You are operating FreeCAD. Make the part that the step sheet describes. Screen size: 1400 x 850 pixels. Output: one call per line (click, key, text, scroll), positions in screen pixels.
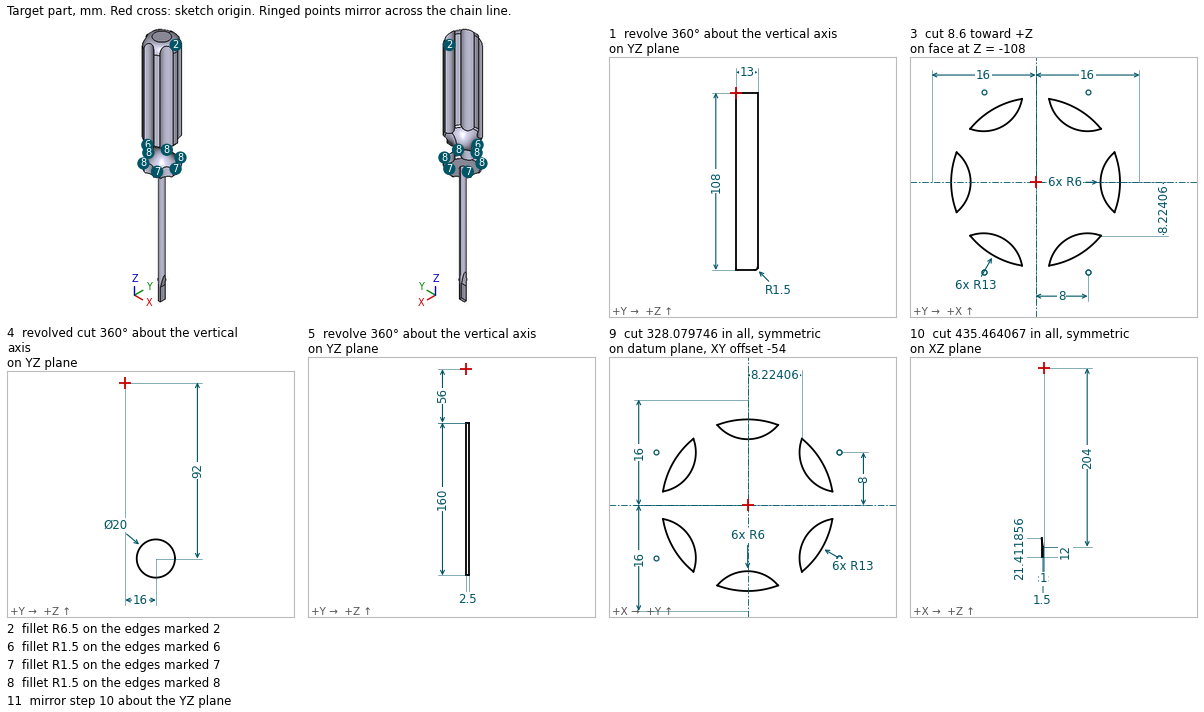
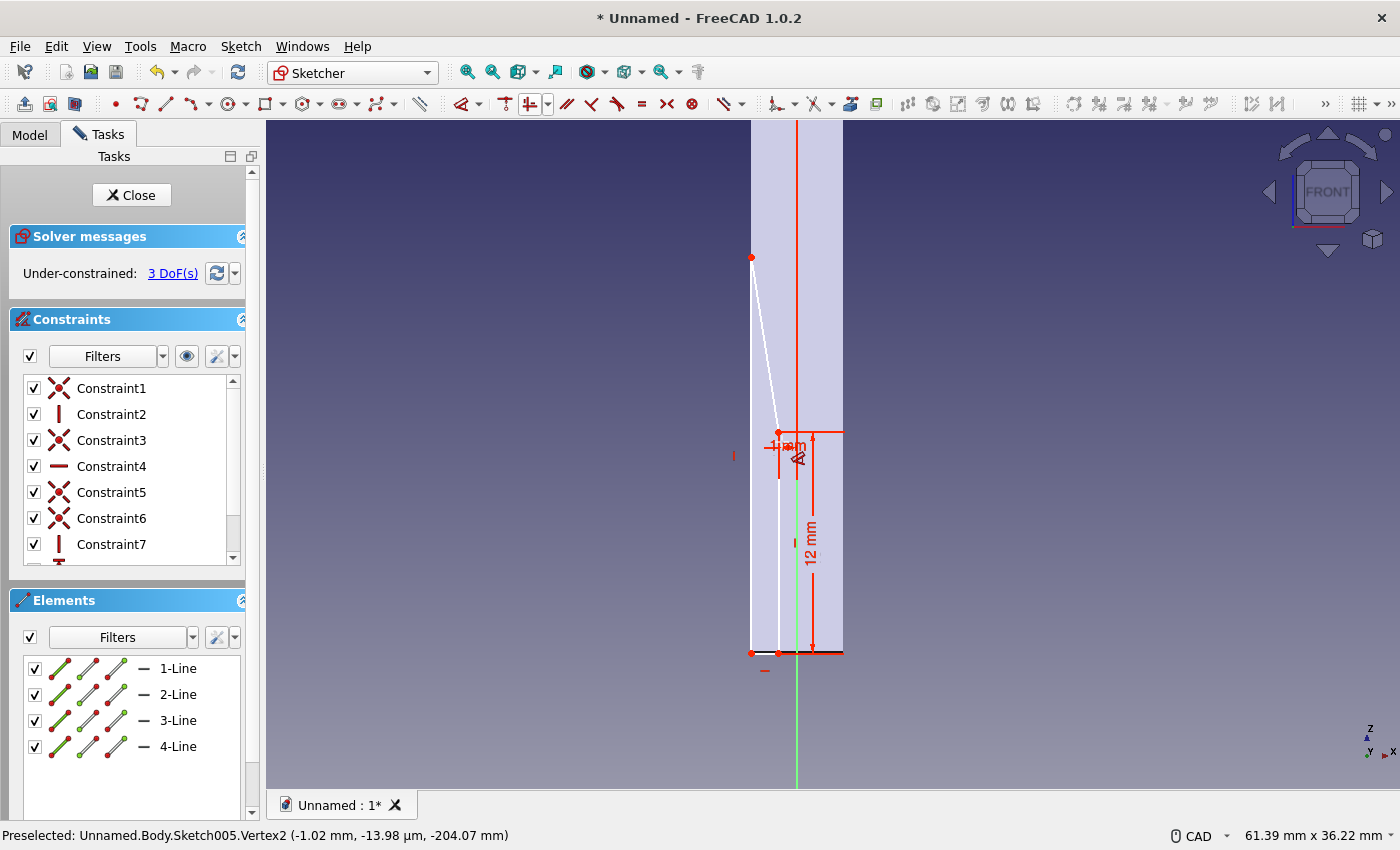
scroll(771, 654, up, 3)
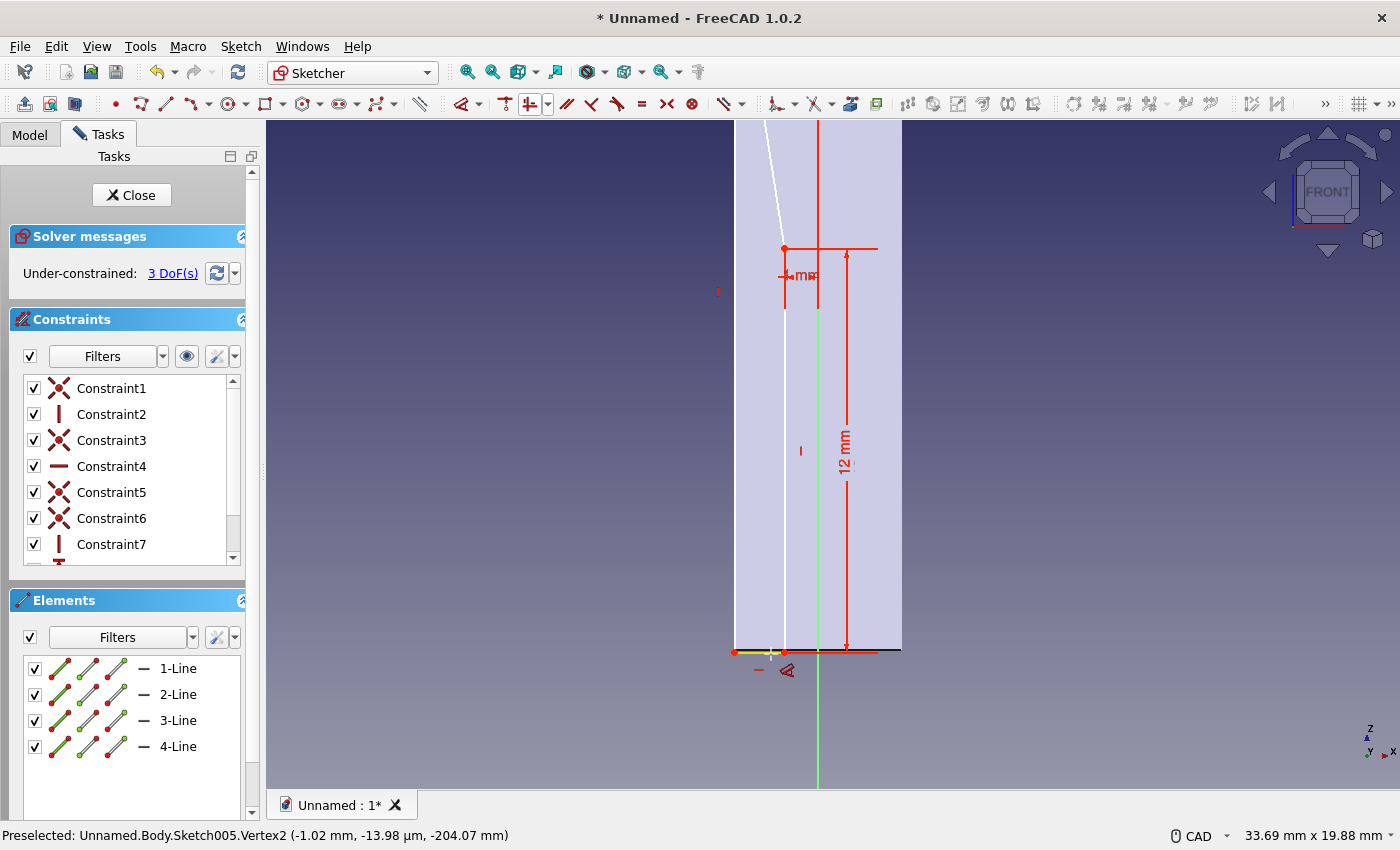
click(770, 653)
click(760, 687)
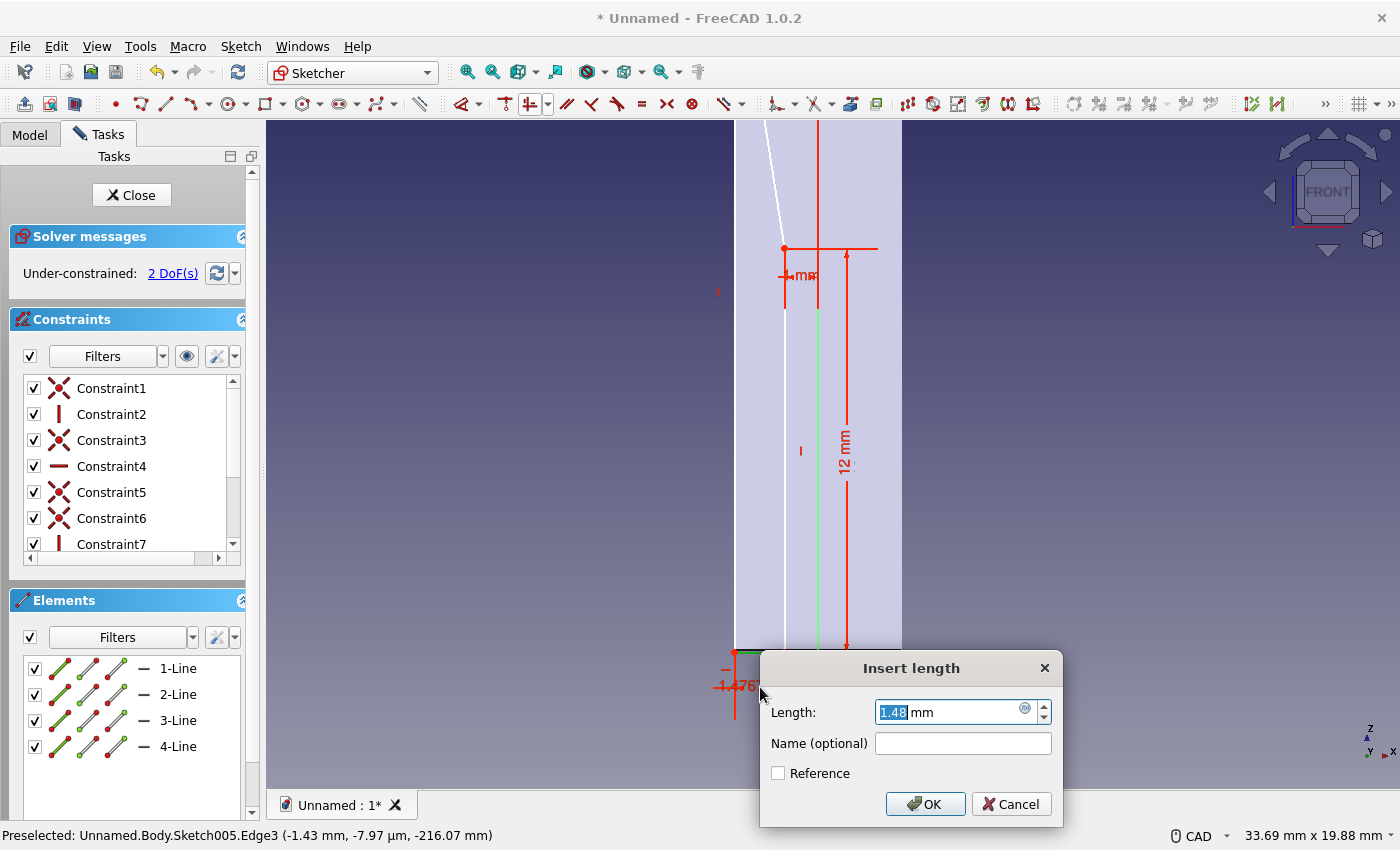
text(1.5)
key(Return)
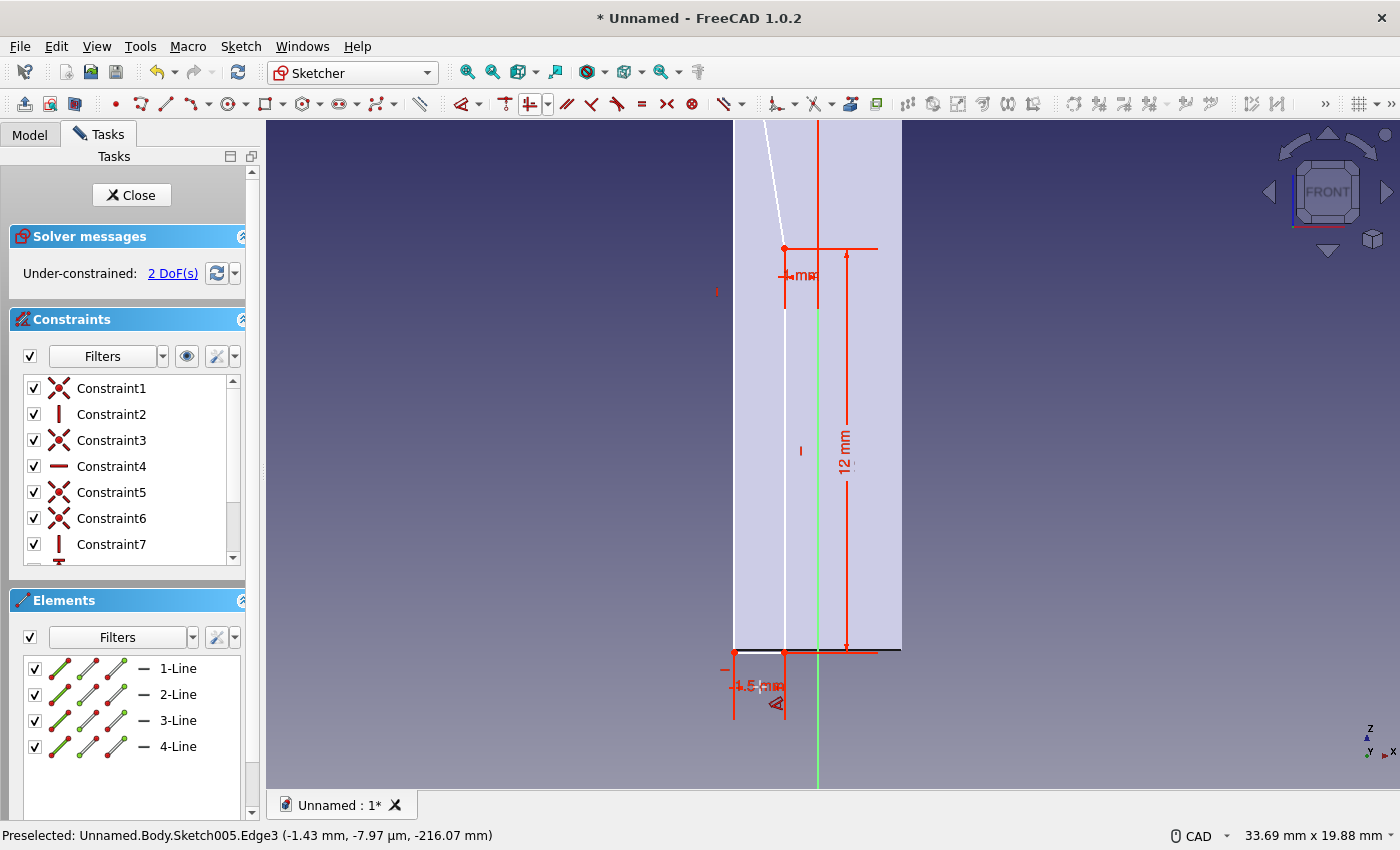
click(785, 249)
click(852, 198)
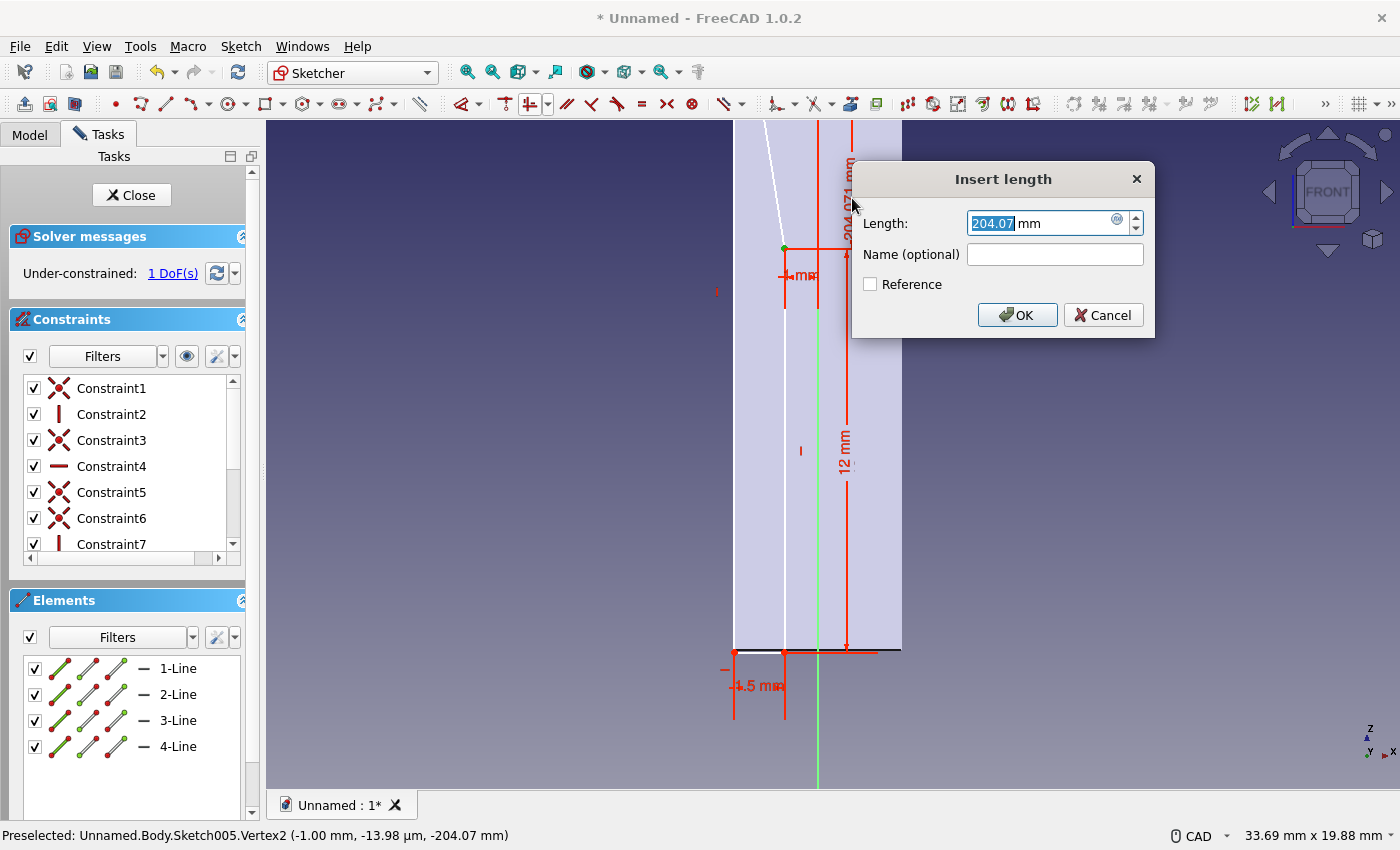
text(204)
key(Return)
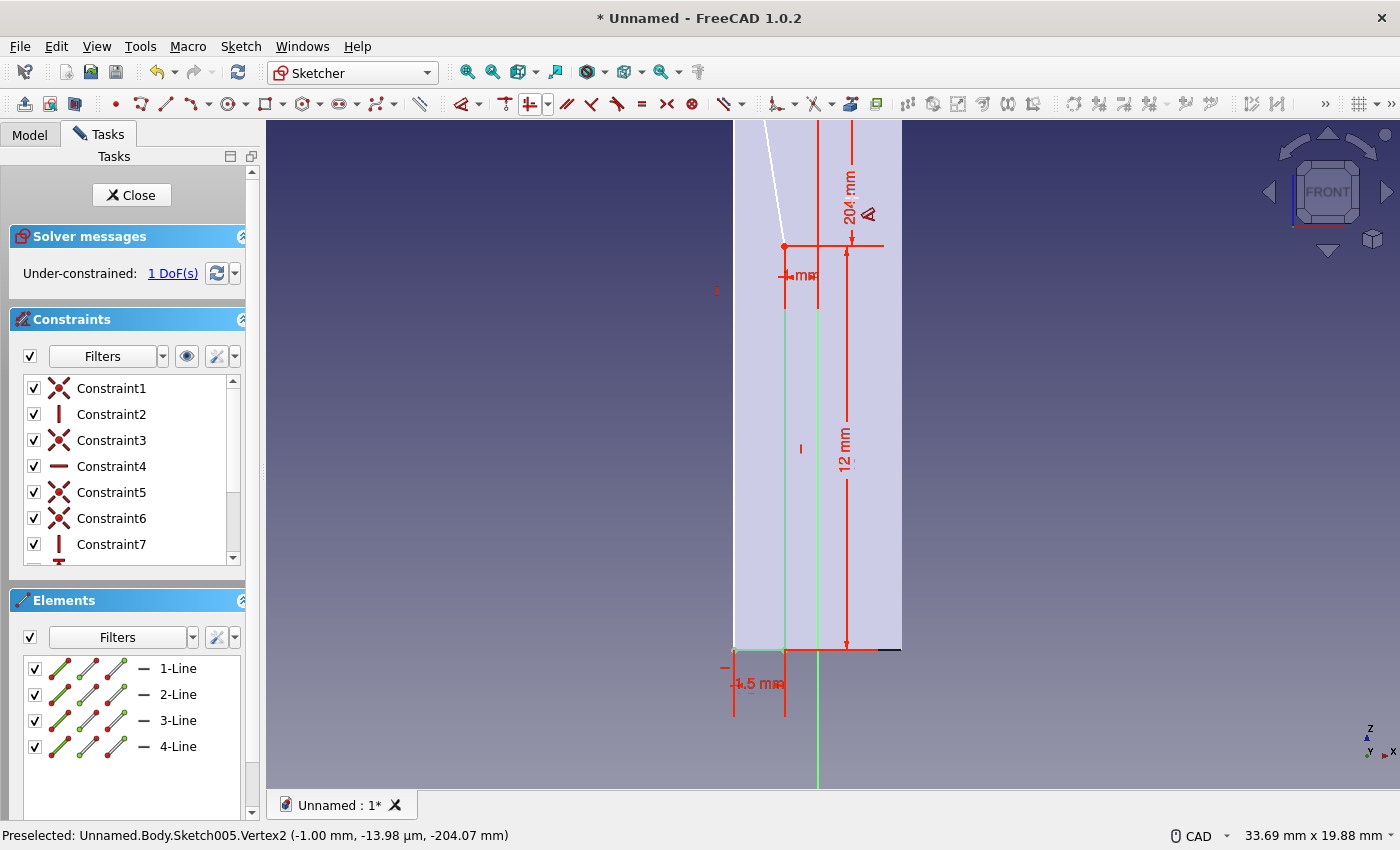
click(734, 435)
click(700, 399)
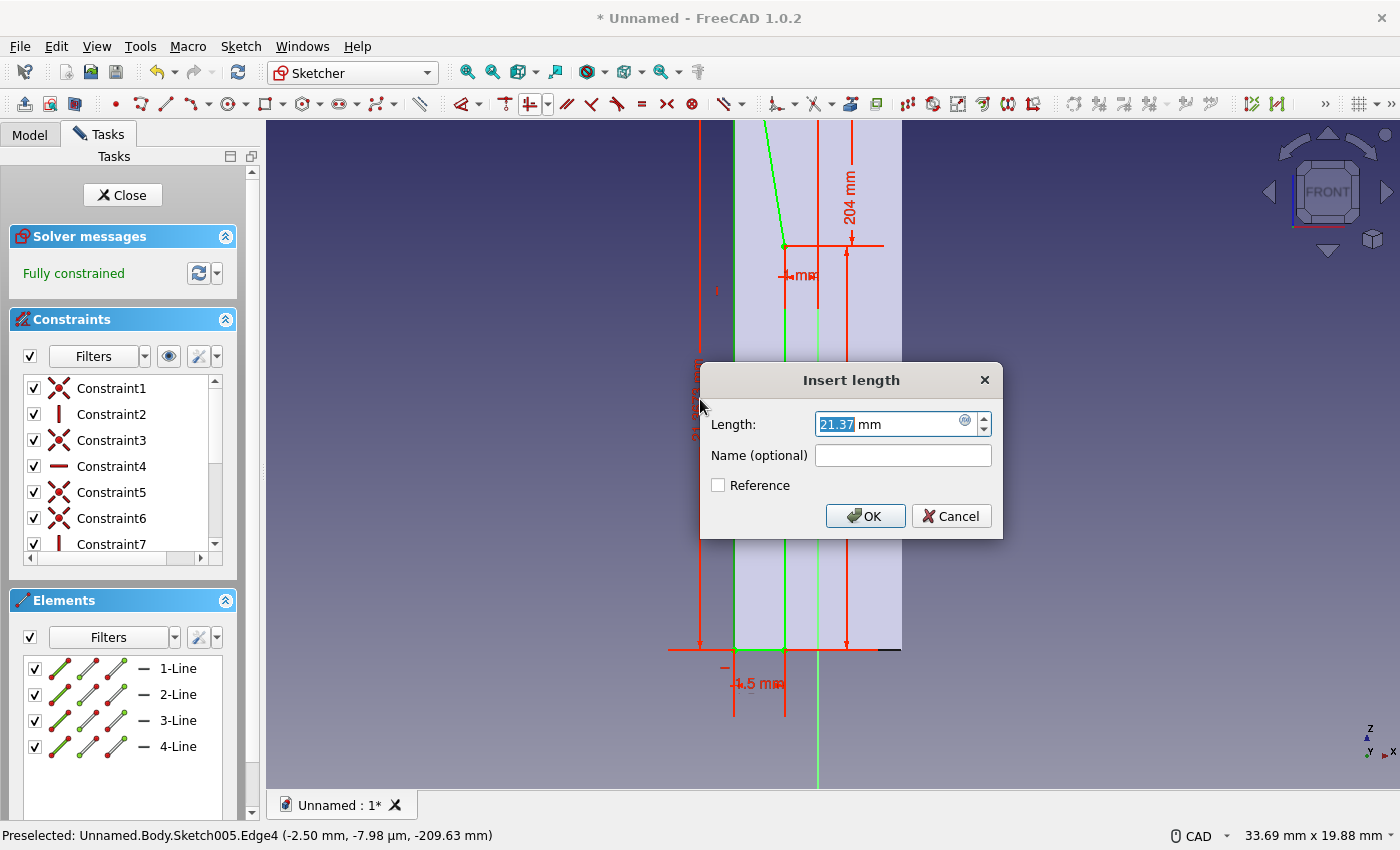
text(21.411856)
key(Return)
key(Escape)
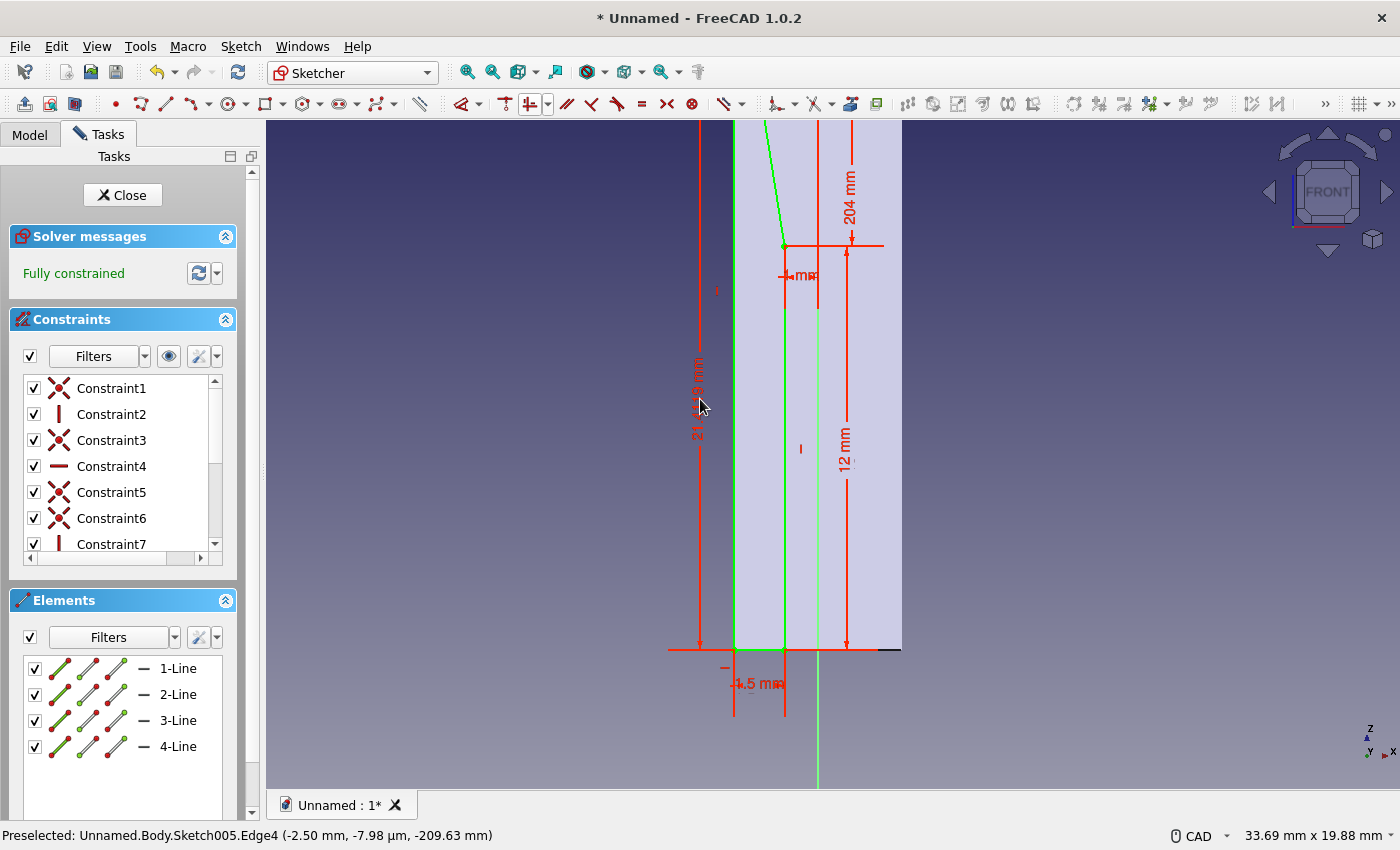
click(123, 195)